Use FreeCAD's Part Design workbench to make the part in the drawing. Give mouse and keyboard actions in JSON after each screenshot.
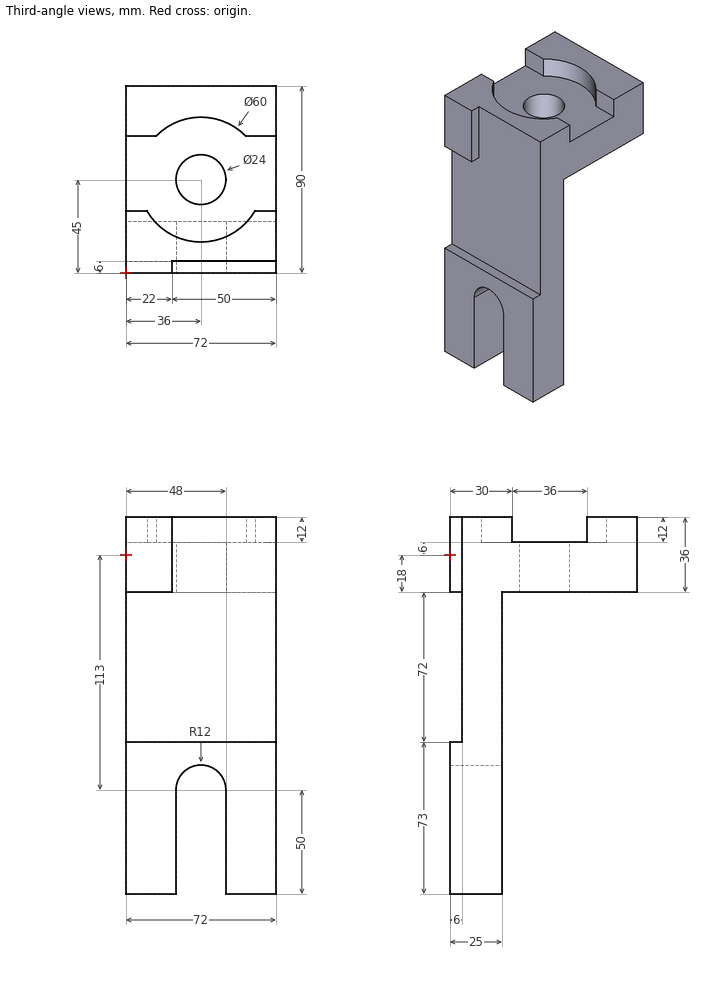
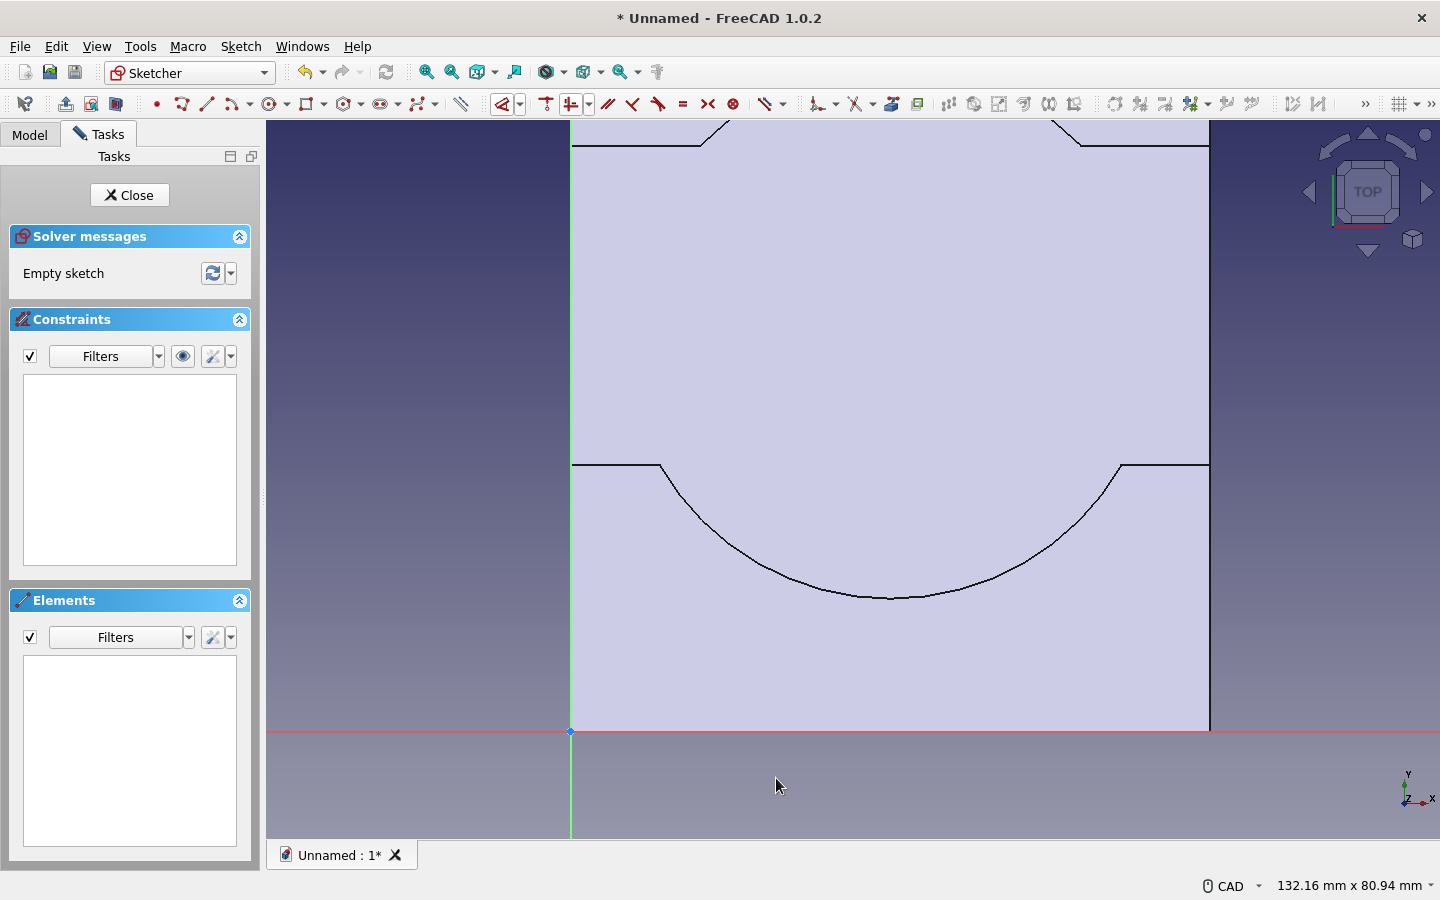
{"action": "key", "text": "g c"}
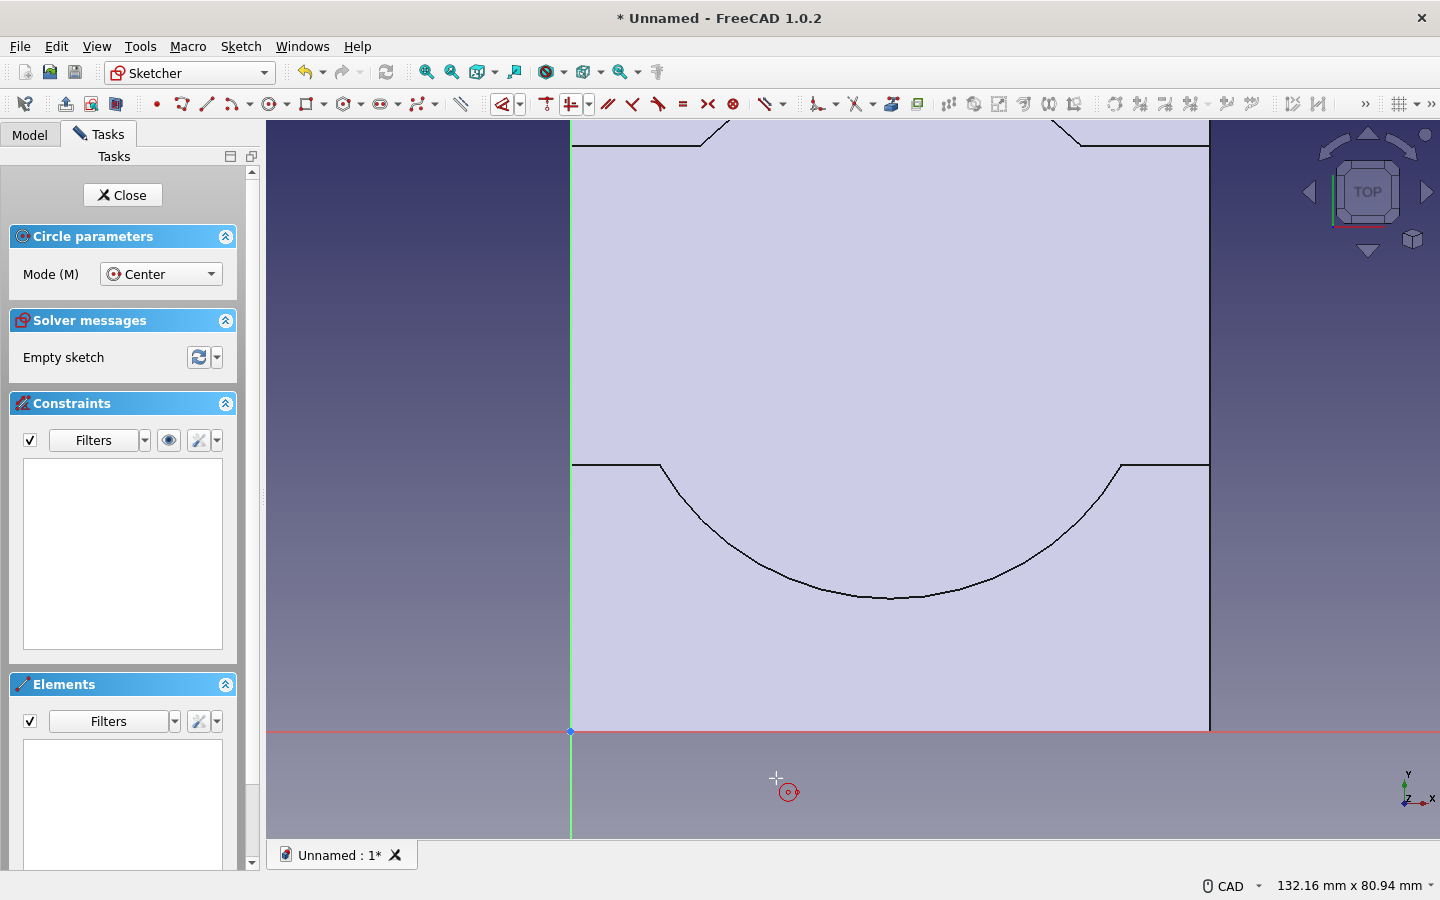
{"action": "left_click", "coordinate": [891, 332]}
{"action": "mouse_move", "coordinate": [966, 257]}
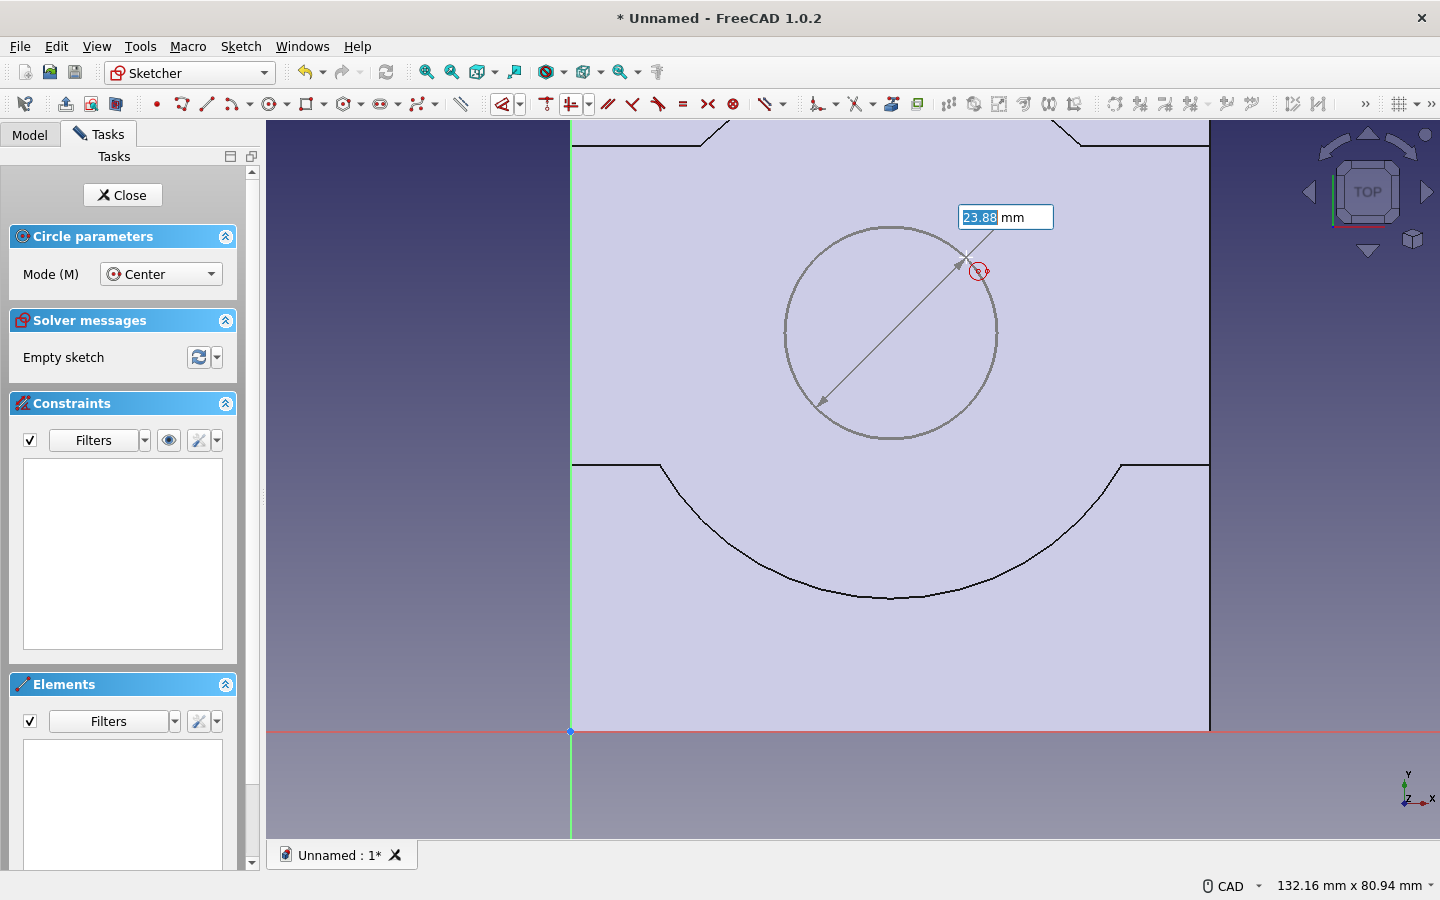
{"action": "type", "text": "24"}
{"action": "key", "text": "Return"}
{"action": "key", "text": "Escape"}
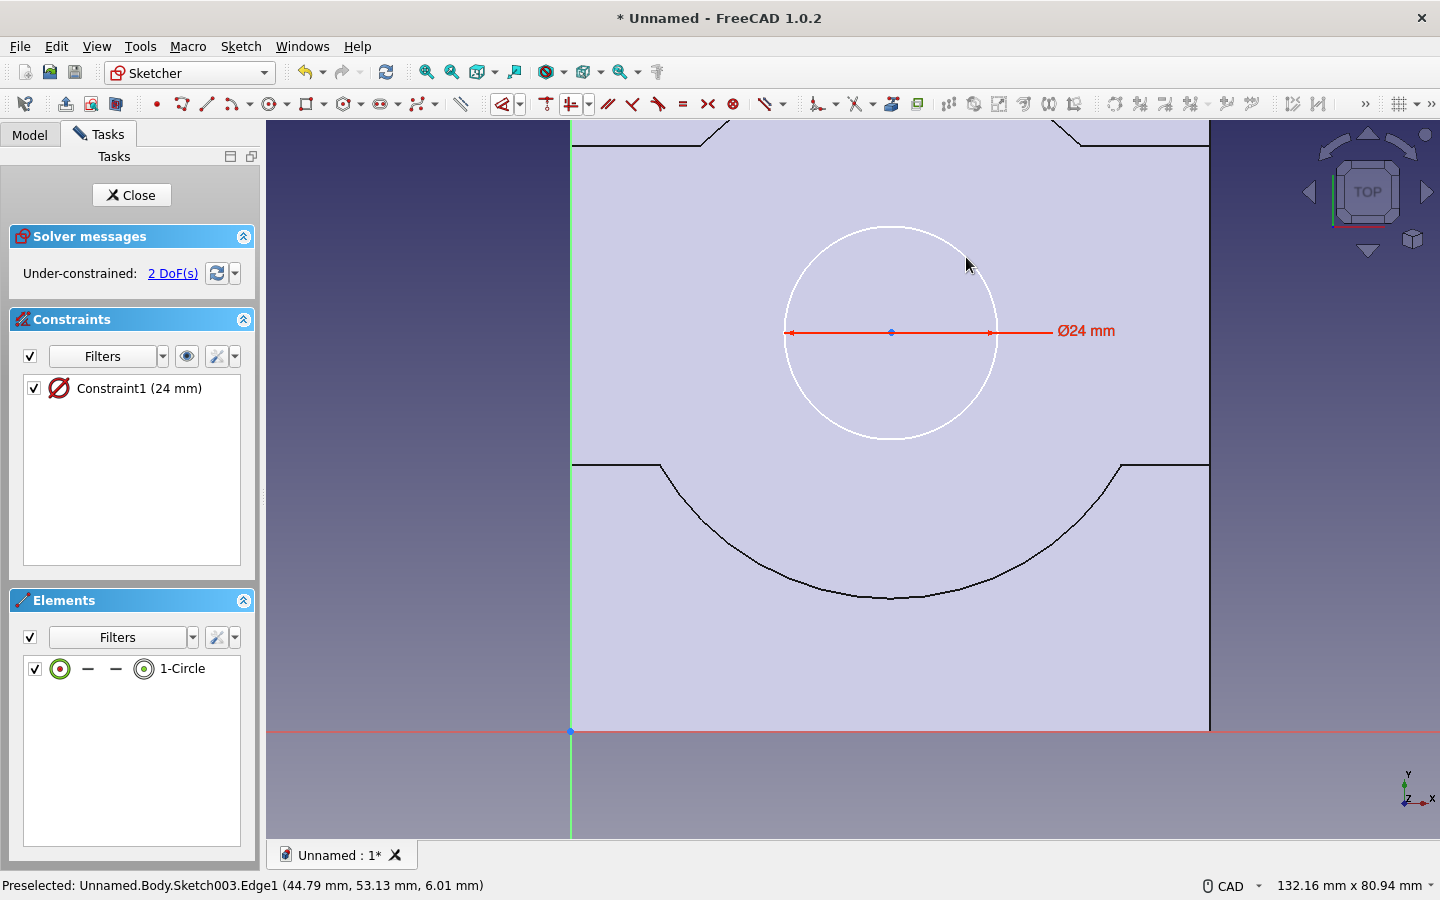
{"action": "left_click", "coordinate": [502, 104]}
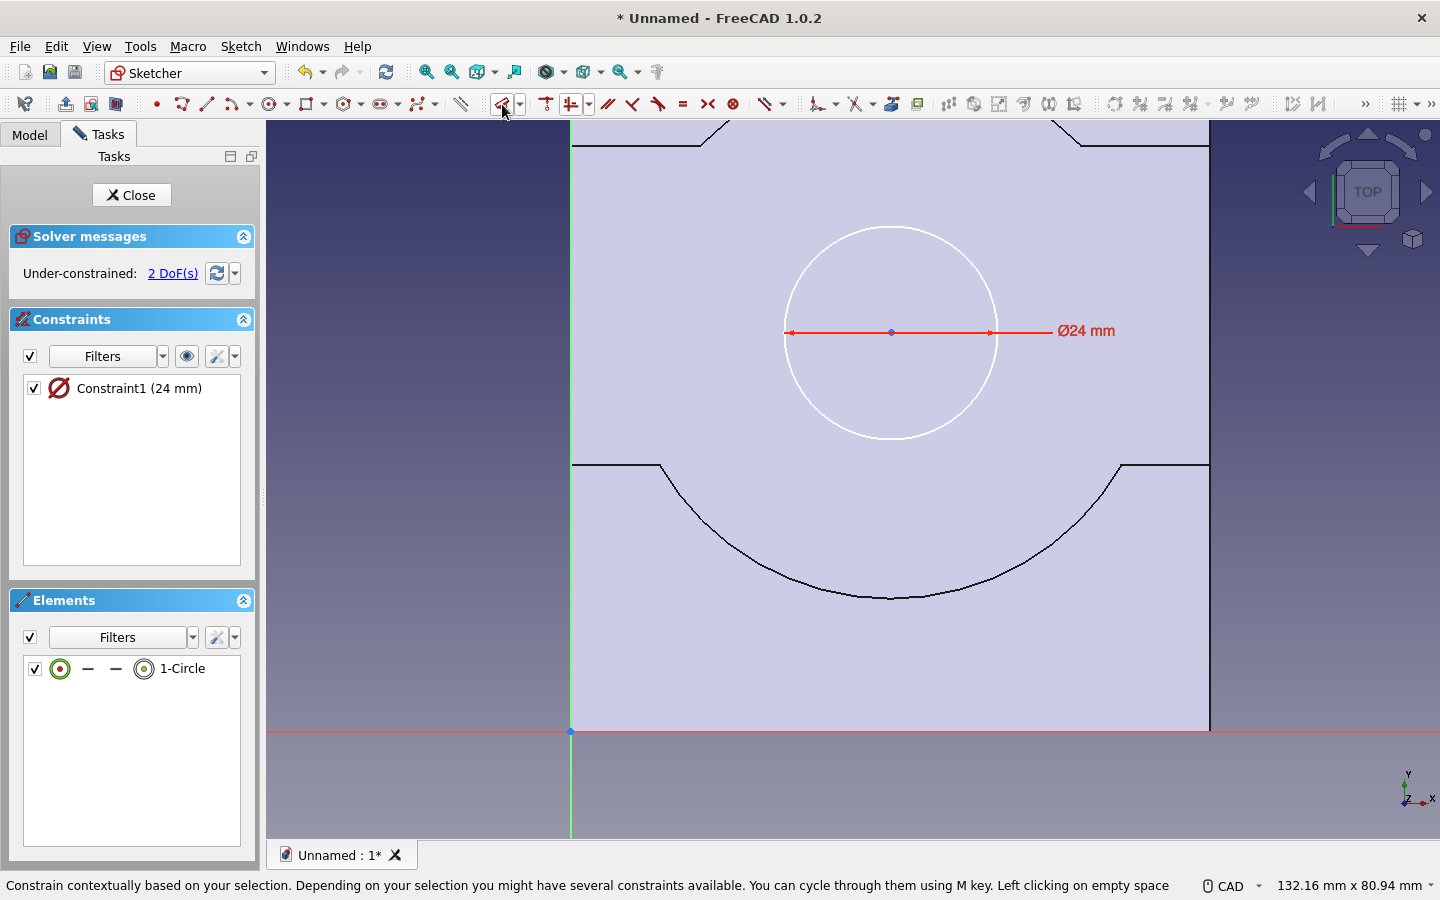
{"action": "left_click", "coordinate": [891, 333]}
{"action": "left_click", "coordinate": [731, 766]}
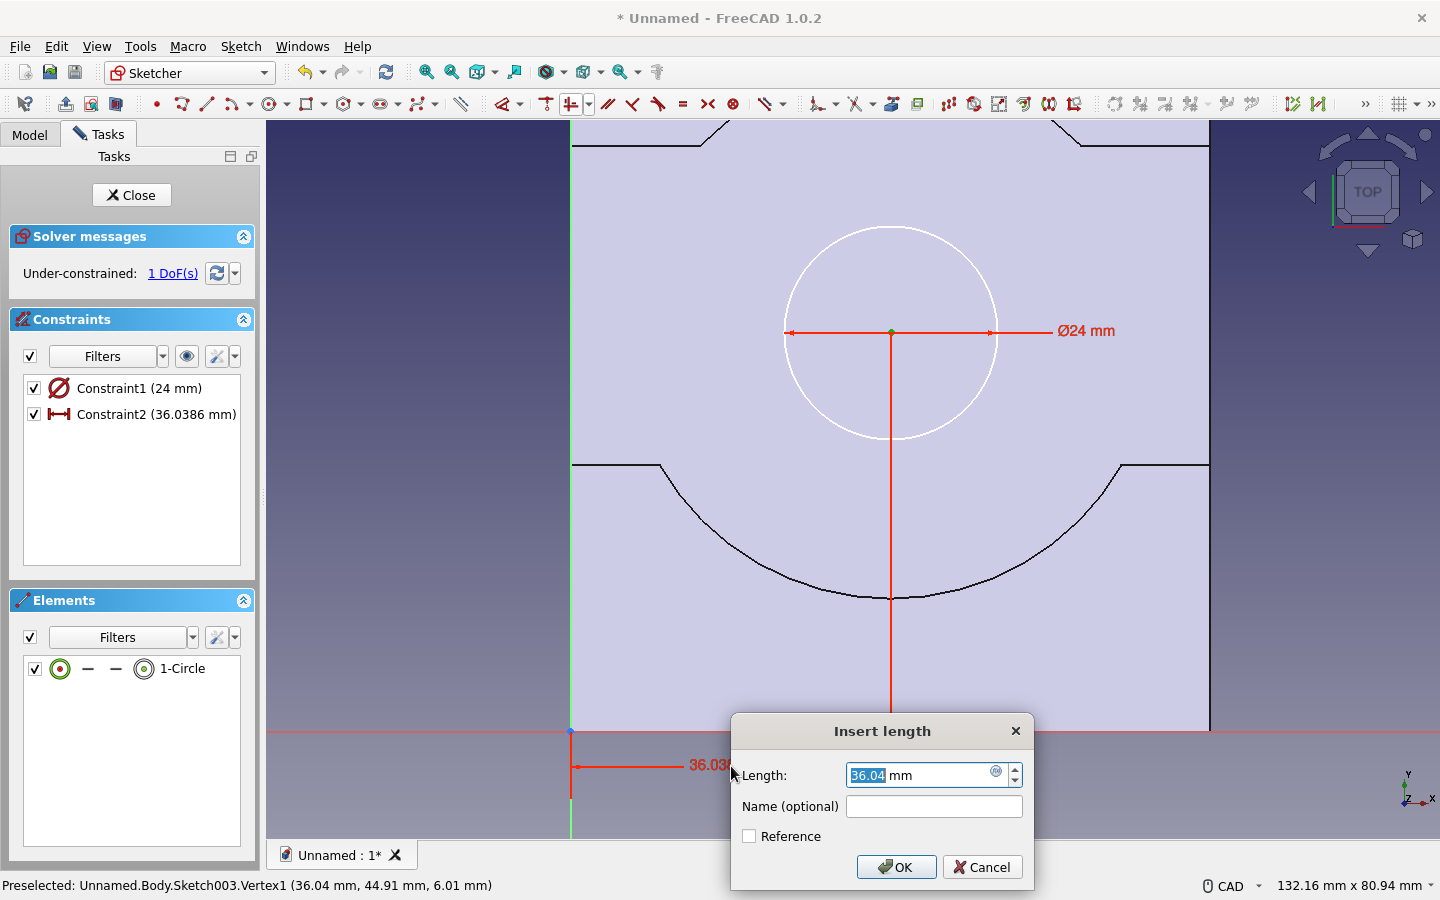
{"action": "type", "text": "36"}
{"action": "key", "text": "Return"}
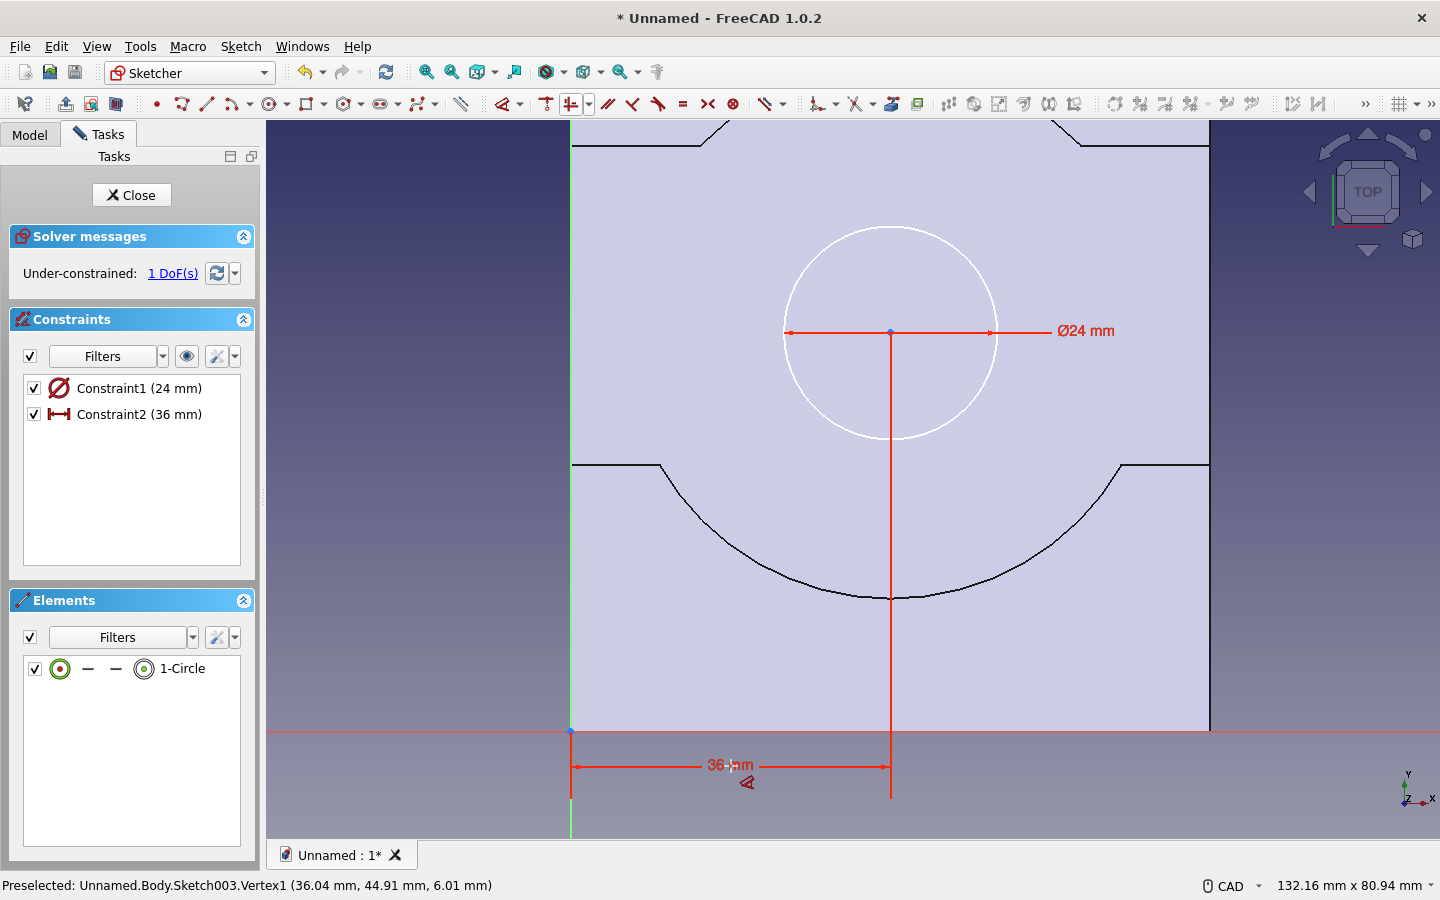
{"action": "left_click", "coordinate": [891, 333]}
{"action": "left_click", "coordinate": [537, 532]}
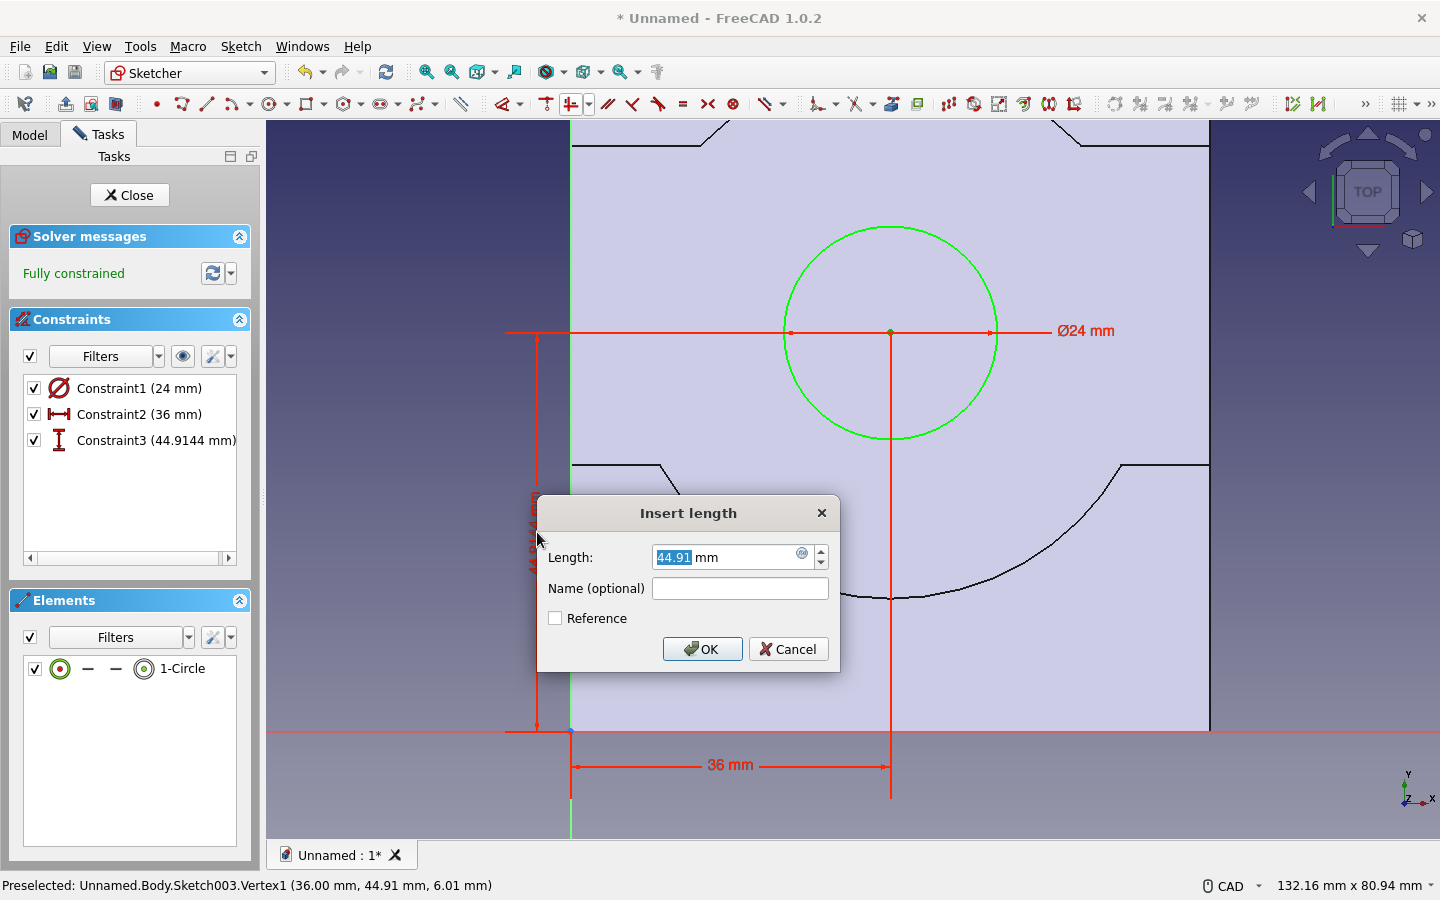
{"action": "type", "text": "45"}
{"action": "key", "text": "Return"}
{"action": "key", "text": "Escape"}